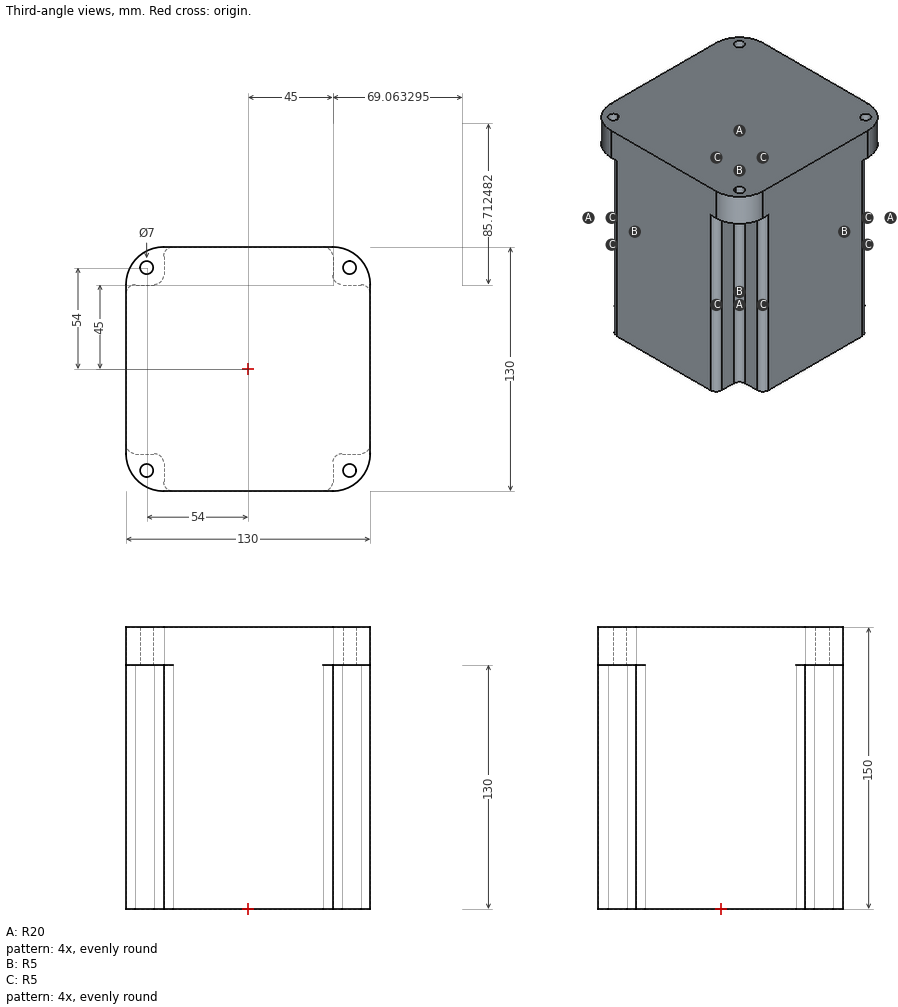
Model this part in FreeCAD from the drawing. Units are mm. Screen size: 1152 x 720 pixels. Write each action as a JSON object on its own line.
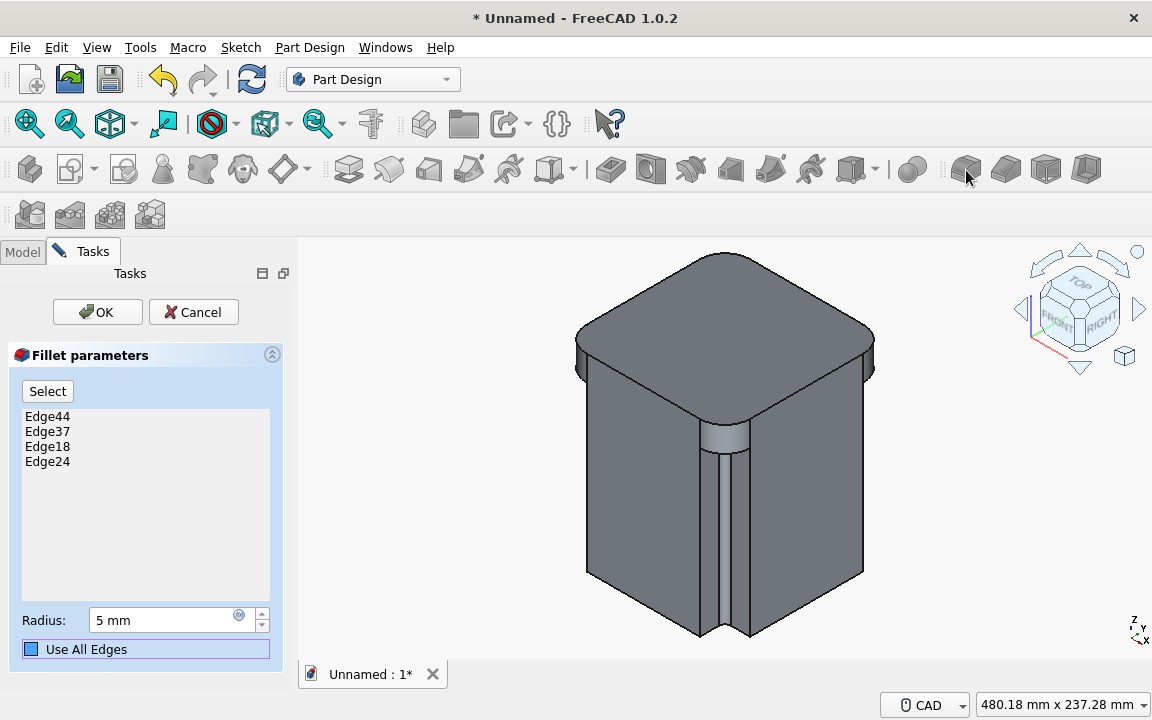
{"action": "left_click", "coordinate": [98, 312]}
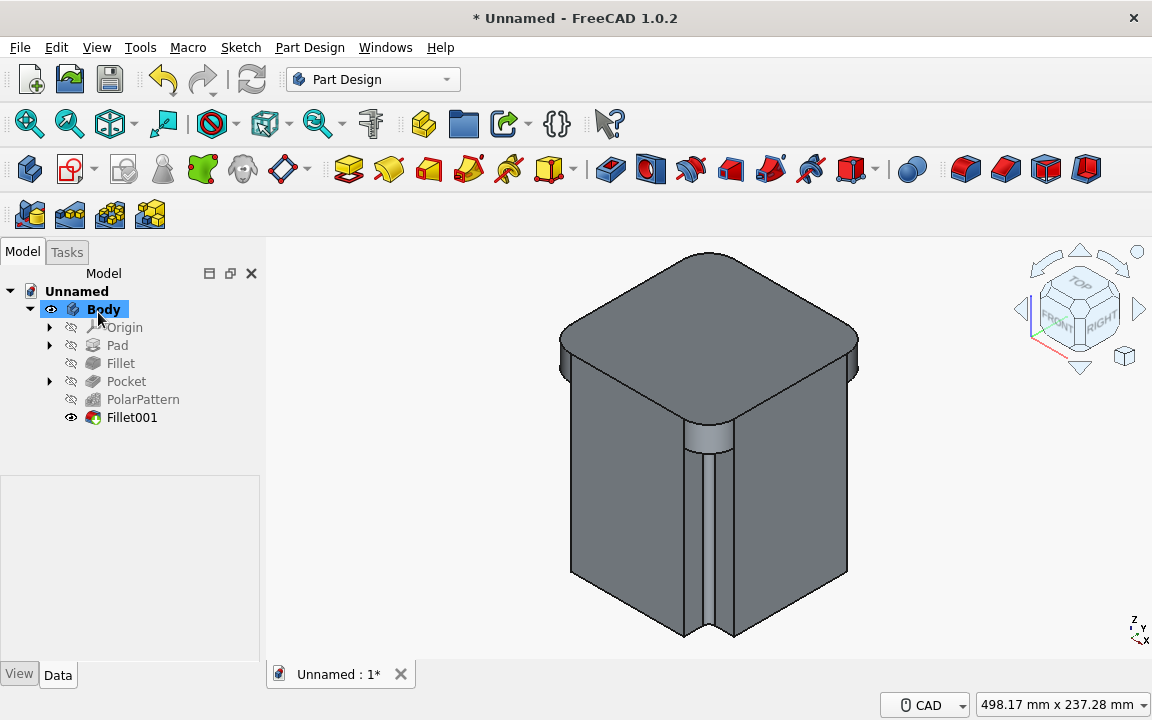
{"action": "left_click", "coordinate": [684, 541]}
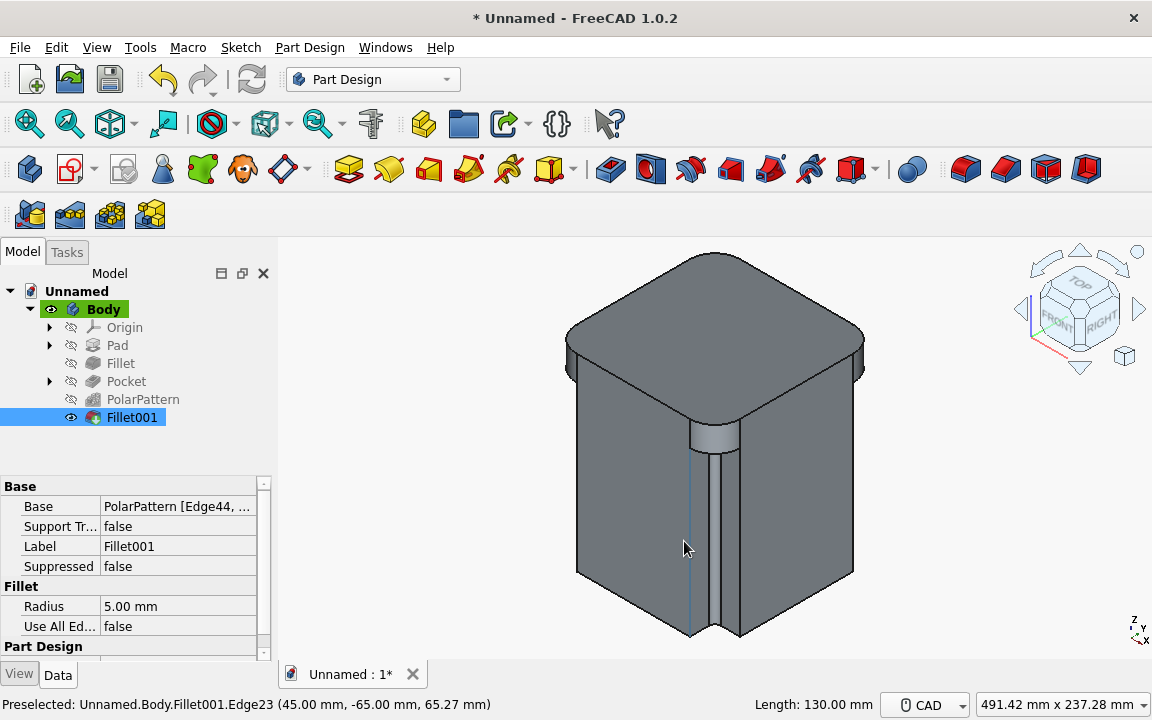
{"action": "left_click", "coordinate": [740, 541], "text": "ctrl"}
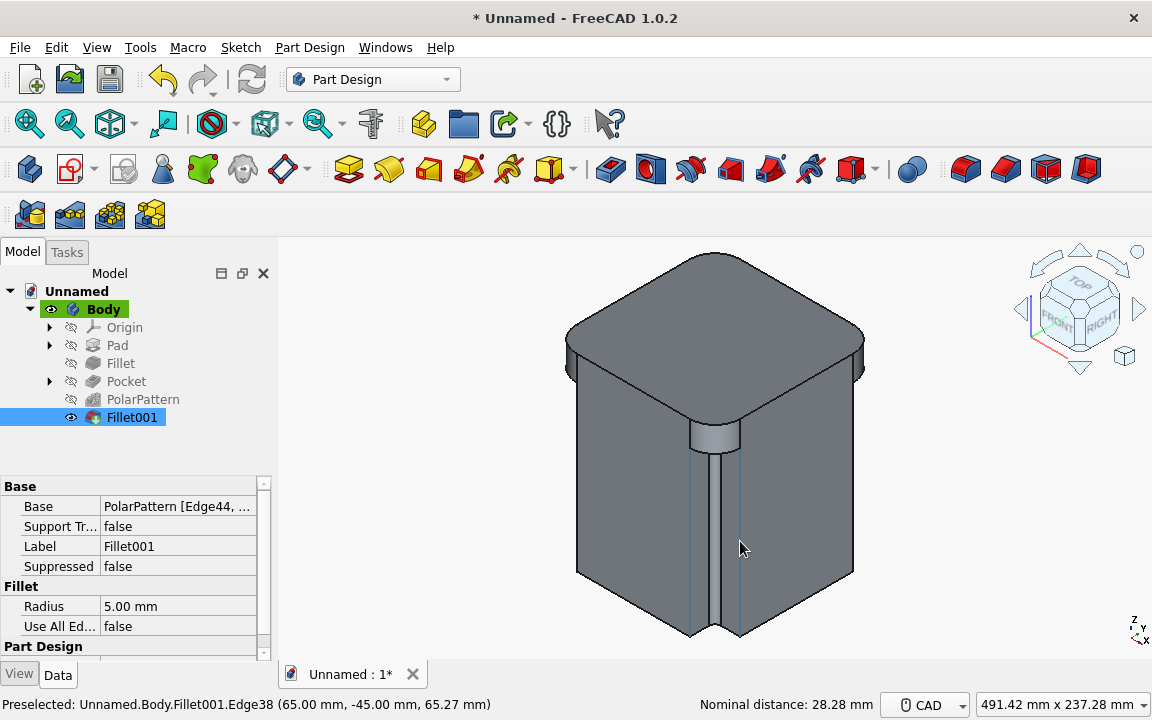
{"action": "key", "text": "2"}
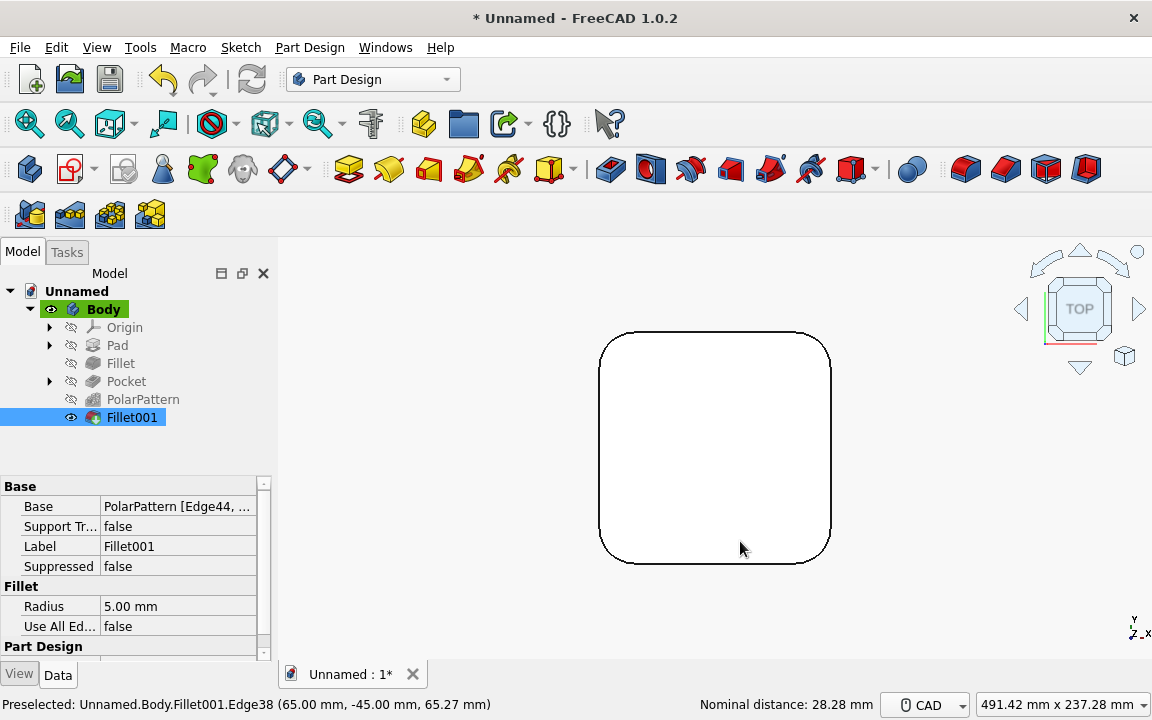
{"action": "key", "text": "0"}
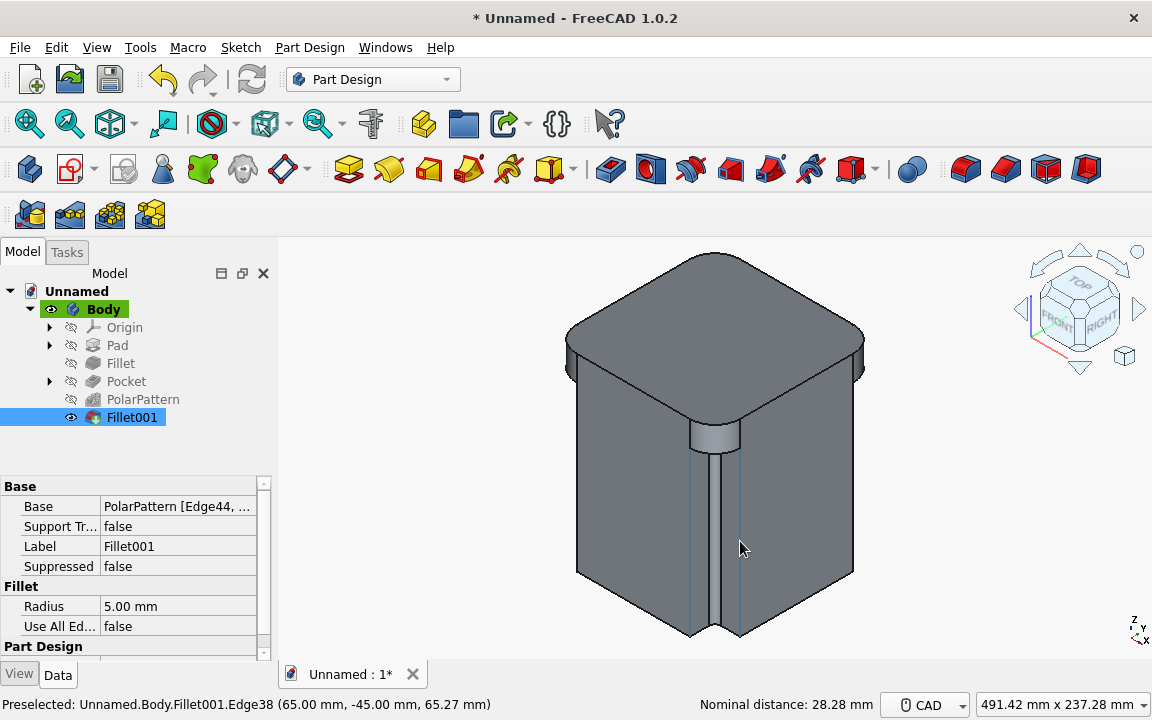
{"action": "key", "text": "1"}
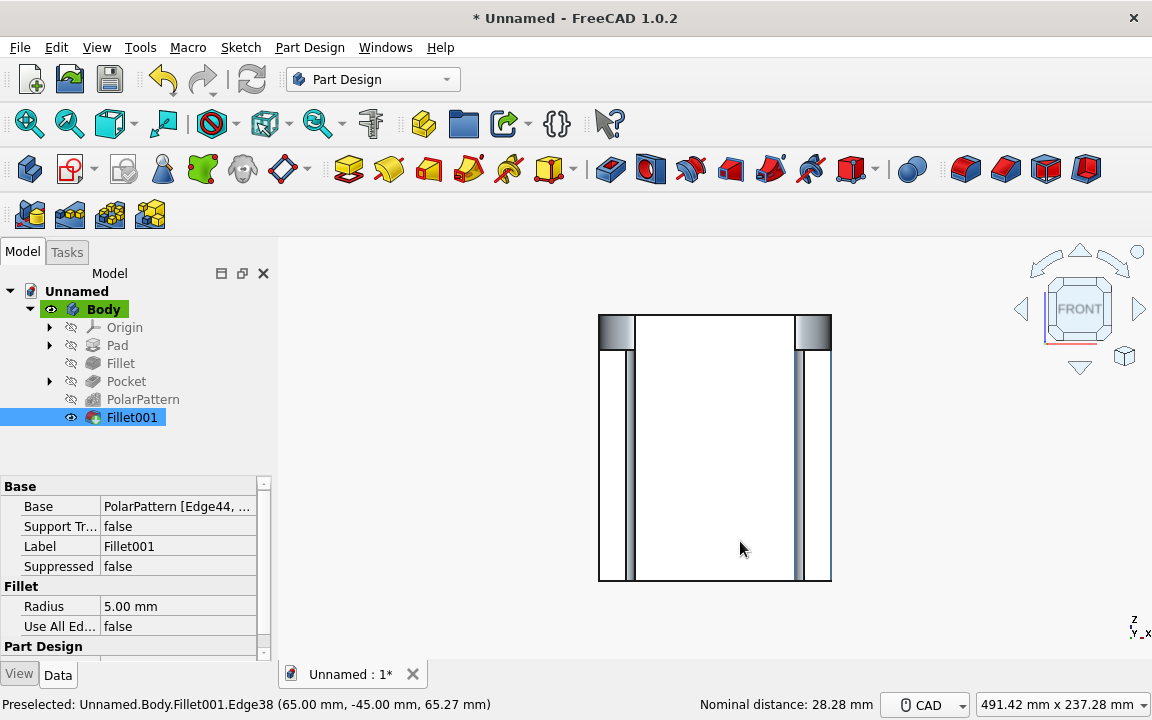
{"action": "left_click", "coordinate": [599, 465], "text": "ctrl"}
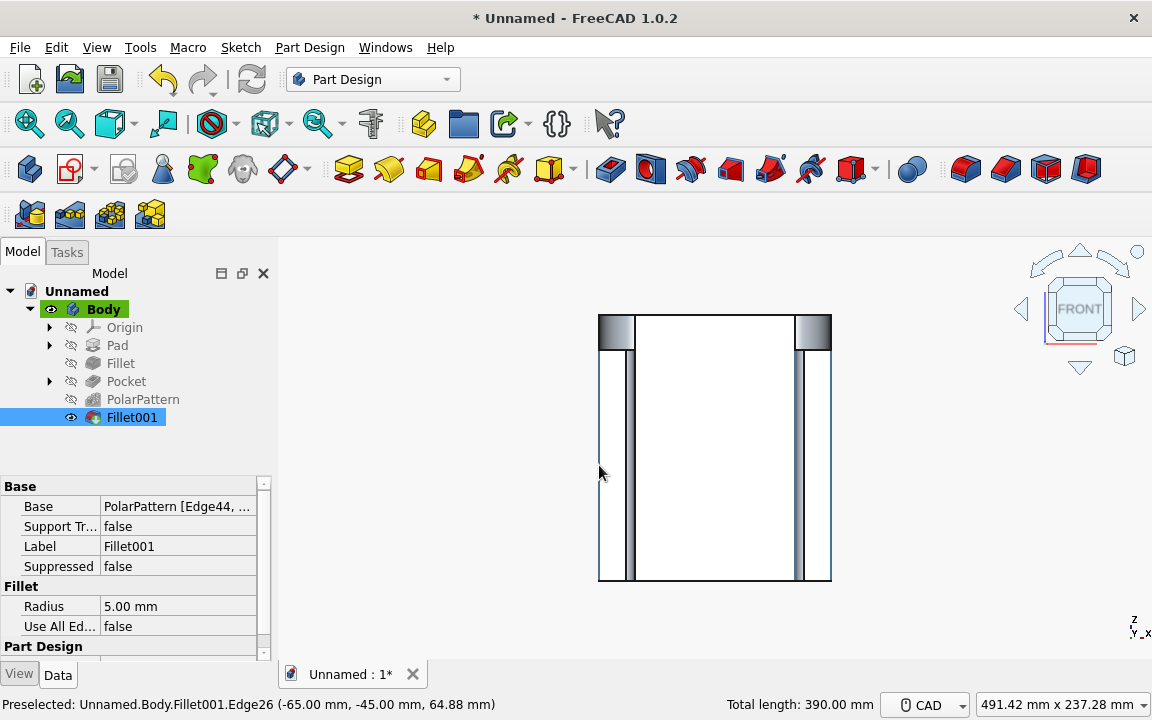
{"action": "left_click", "coordinate": [635, 465], "text": "ctrl"}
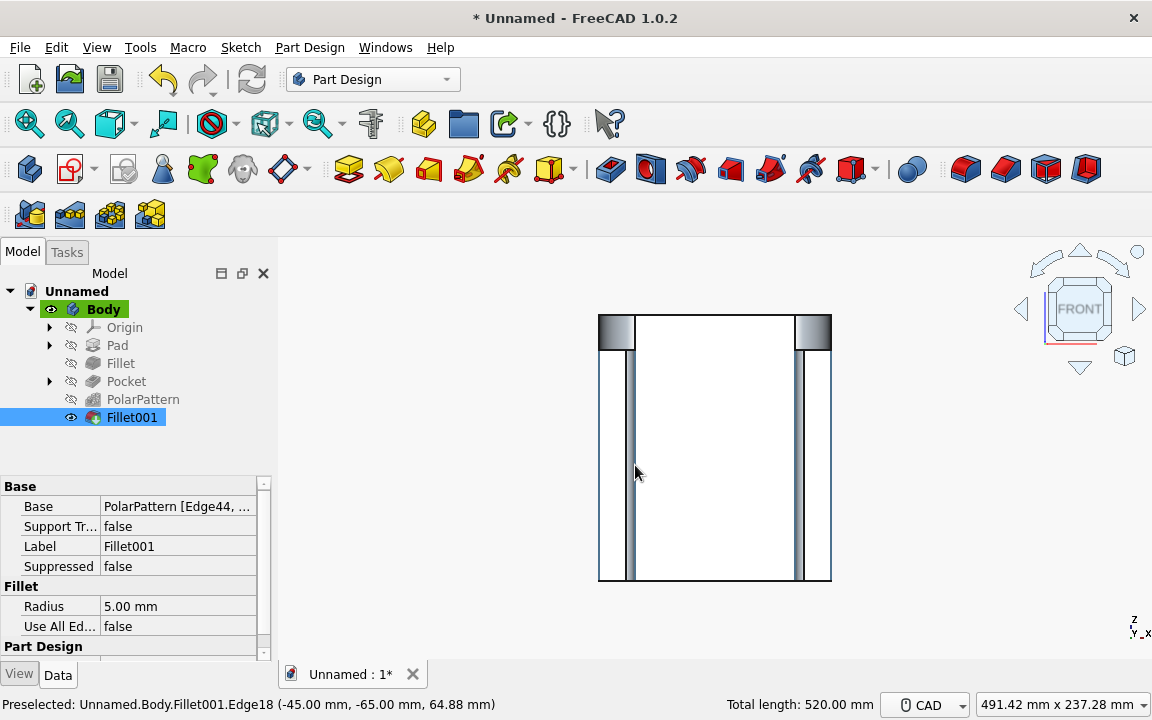
{"action": "key", "text": "3"}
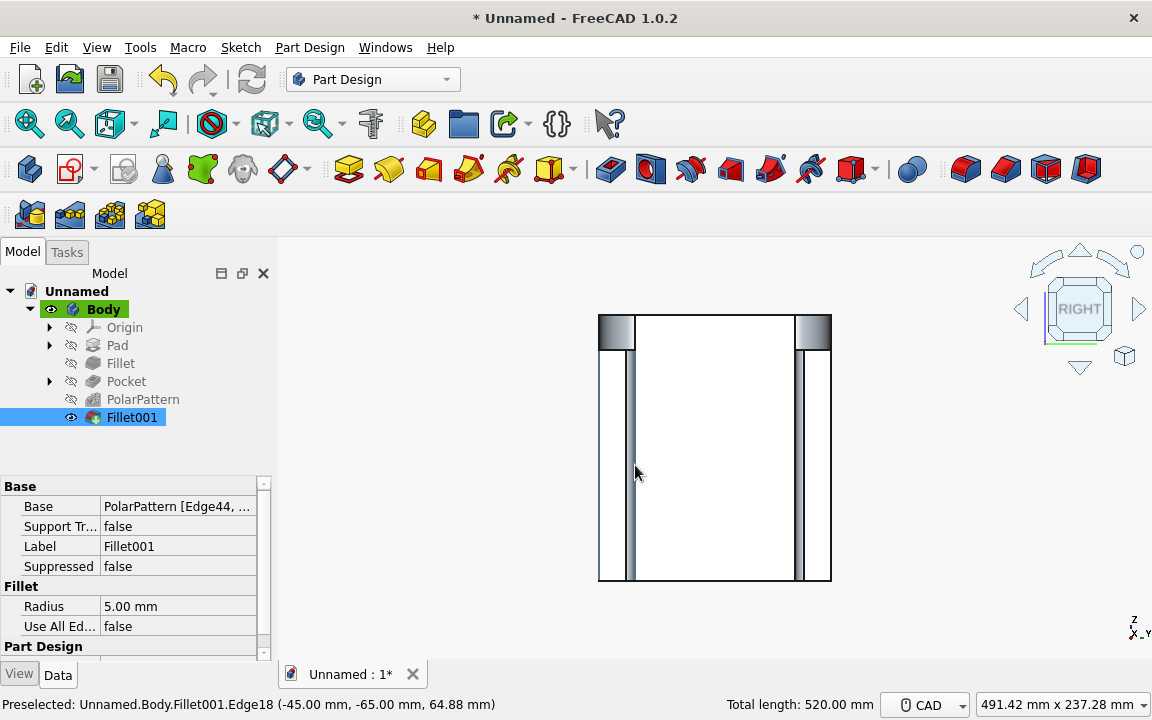
{"action": "left_click", "coordinate": [795, 465], "text": "ctrl"}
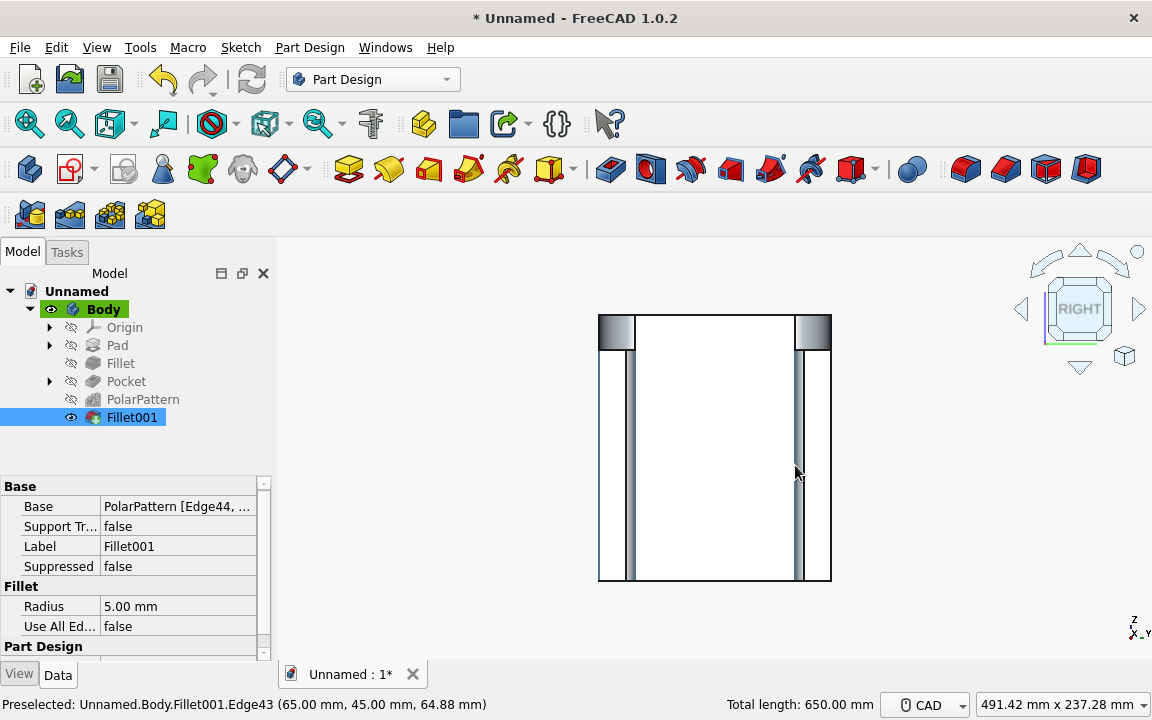
{"action": "left_click", "coordinate": [831, 465], "text": "ctrl"}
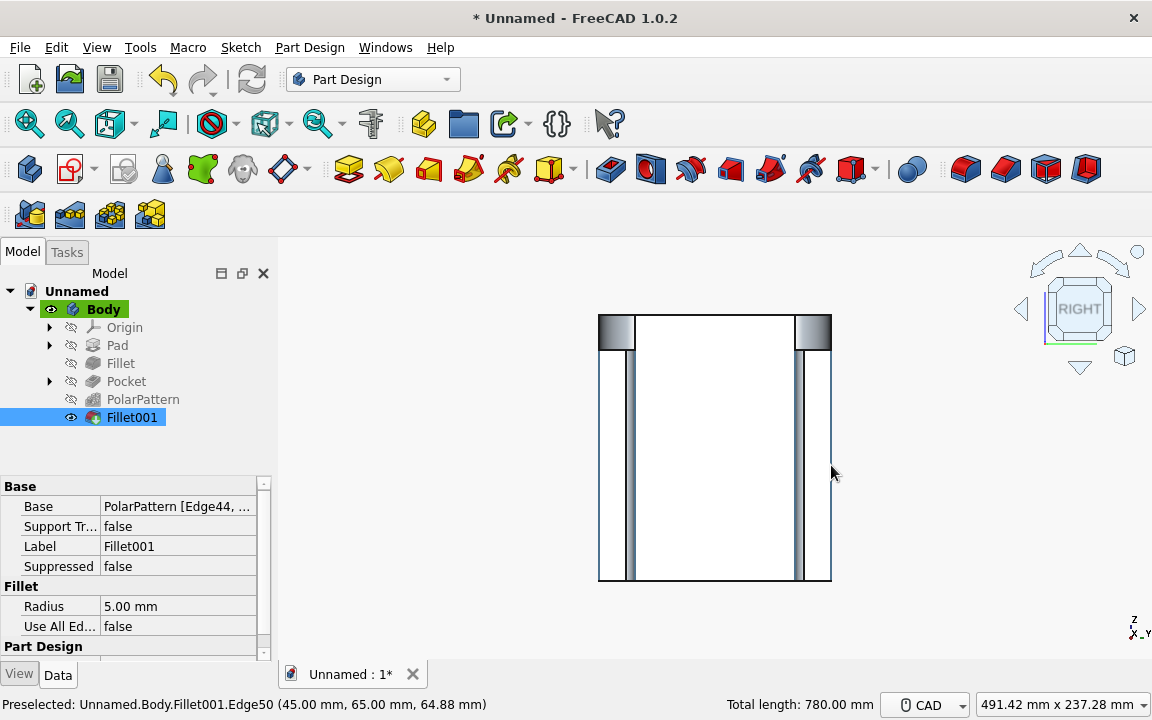
{"action": "key", "text": "5"}